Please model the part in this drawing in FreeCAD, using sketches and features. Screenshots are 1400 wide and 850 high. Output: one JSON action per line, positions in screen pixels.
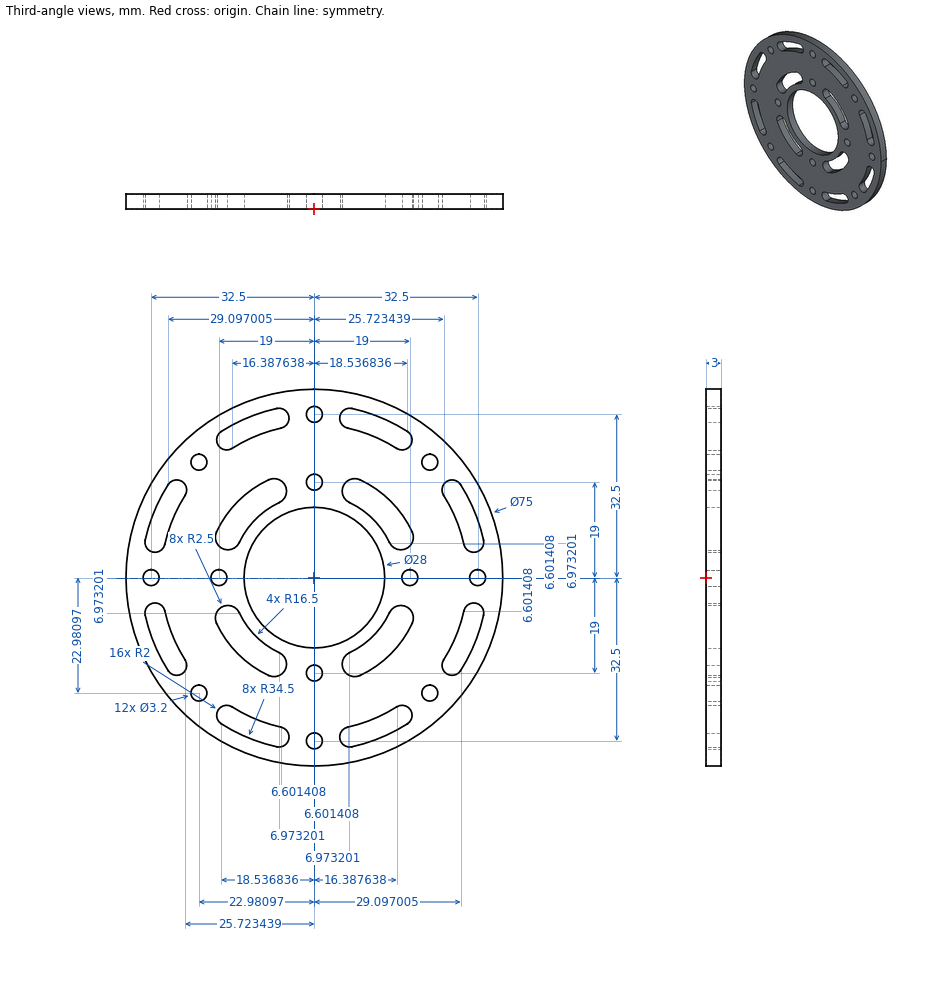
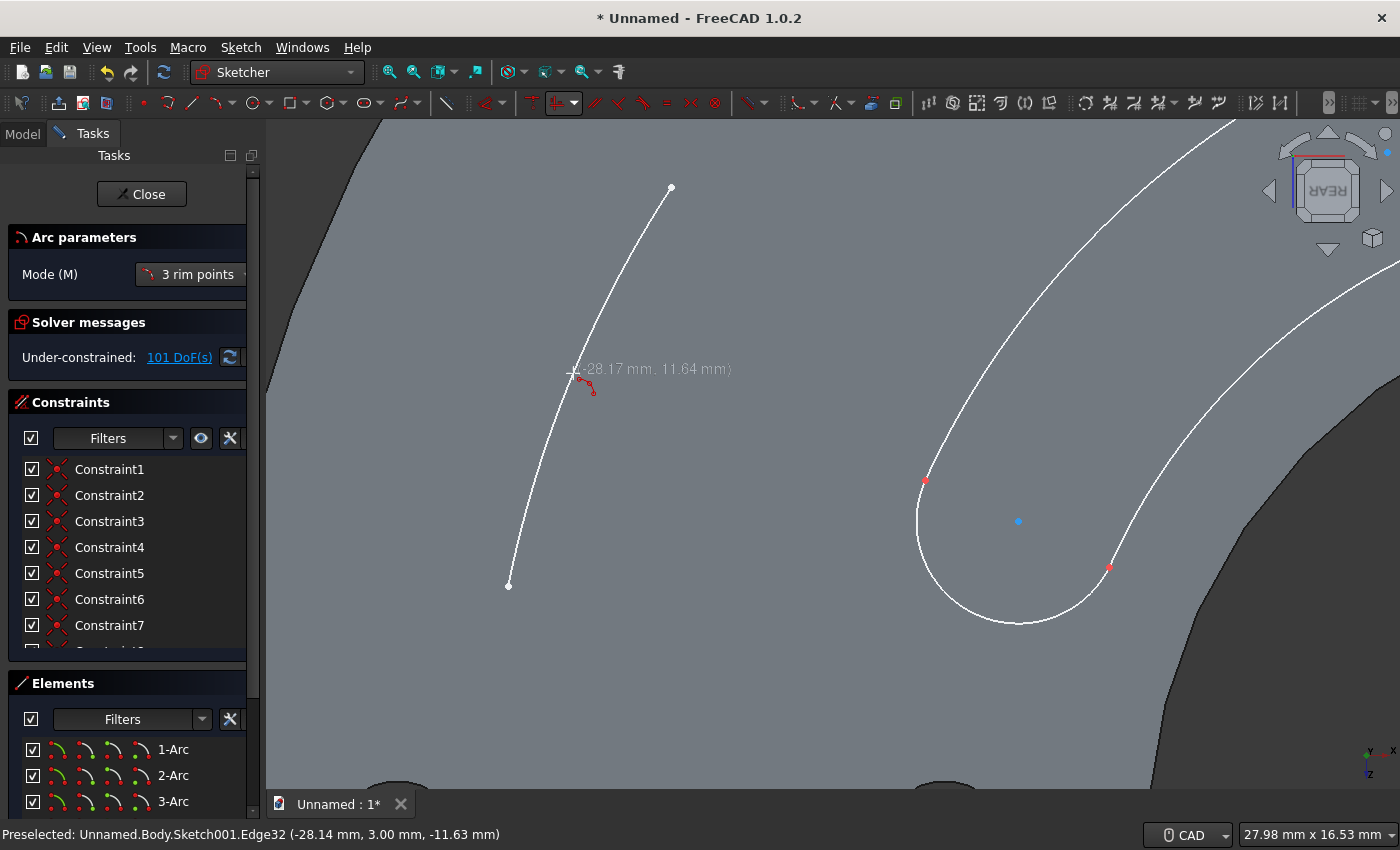
{"action": "scroll", "coordinate": [576, 376], "scroll_direction": "down", "scroll_amount": 9}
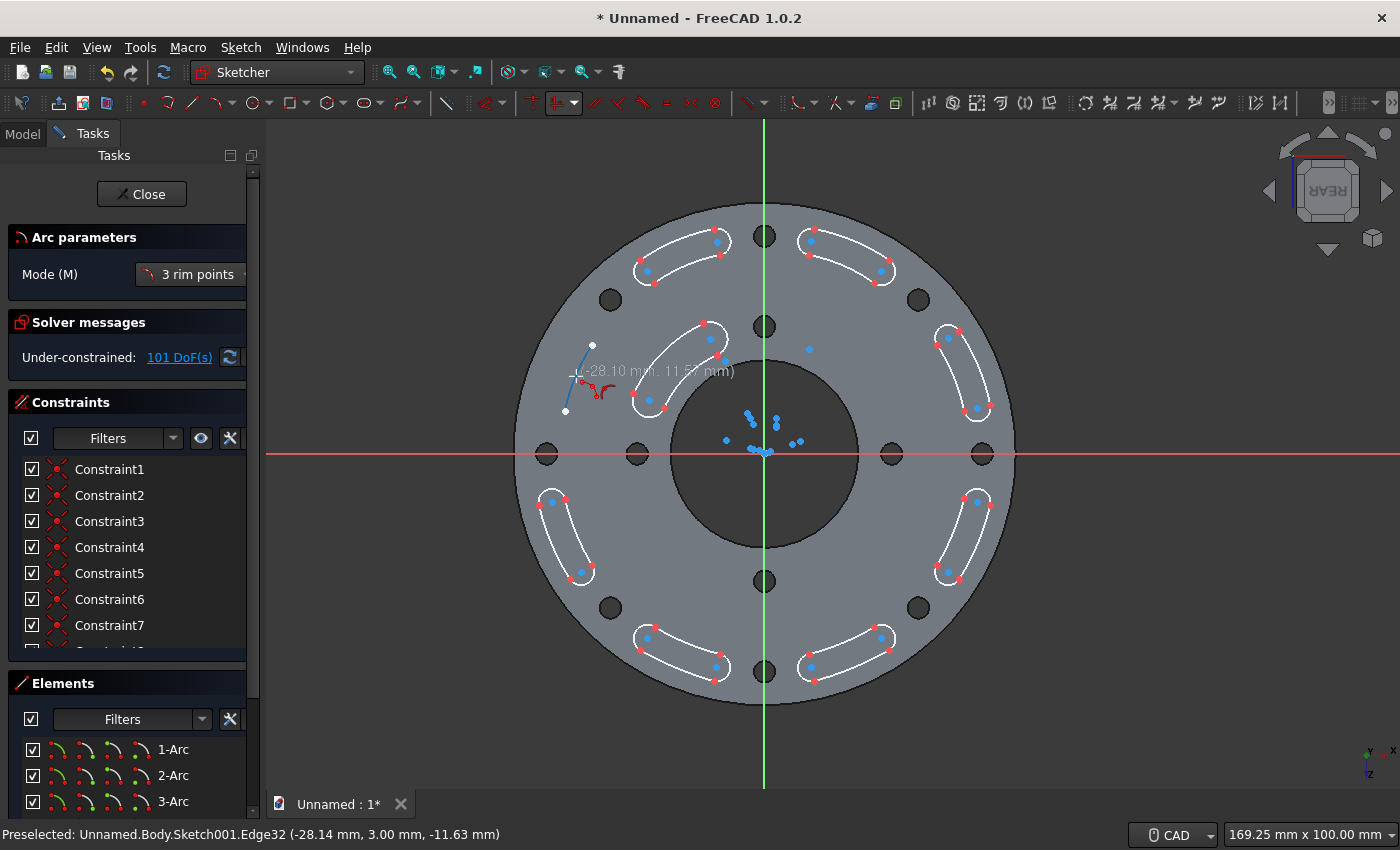
{"action": "left_click", "coordinate": [592, 345]}
{"action": "left_click", "coordinate": [570, 330]}
{"action": "left_click", "coordinate": [588, 326]}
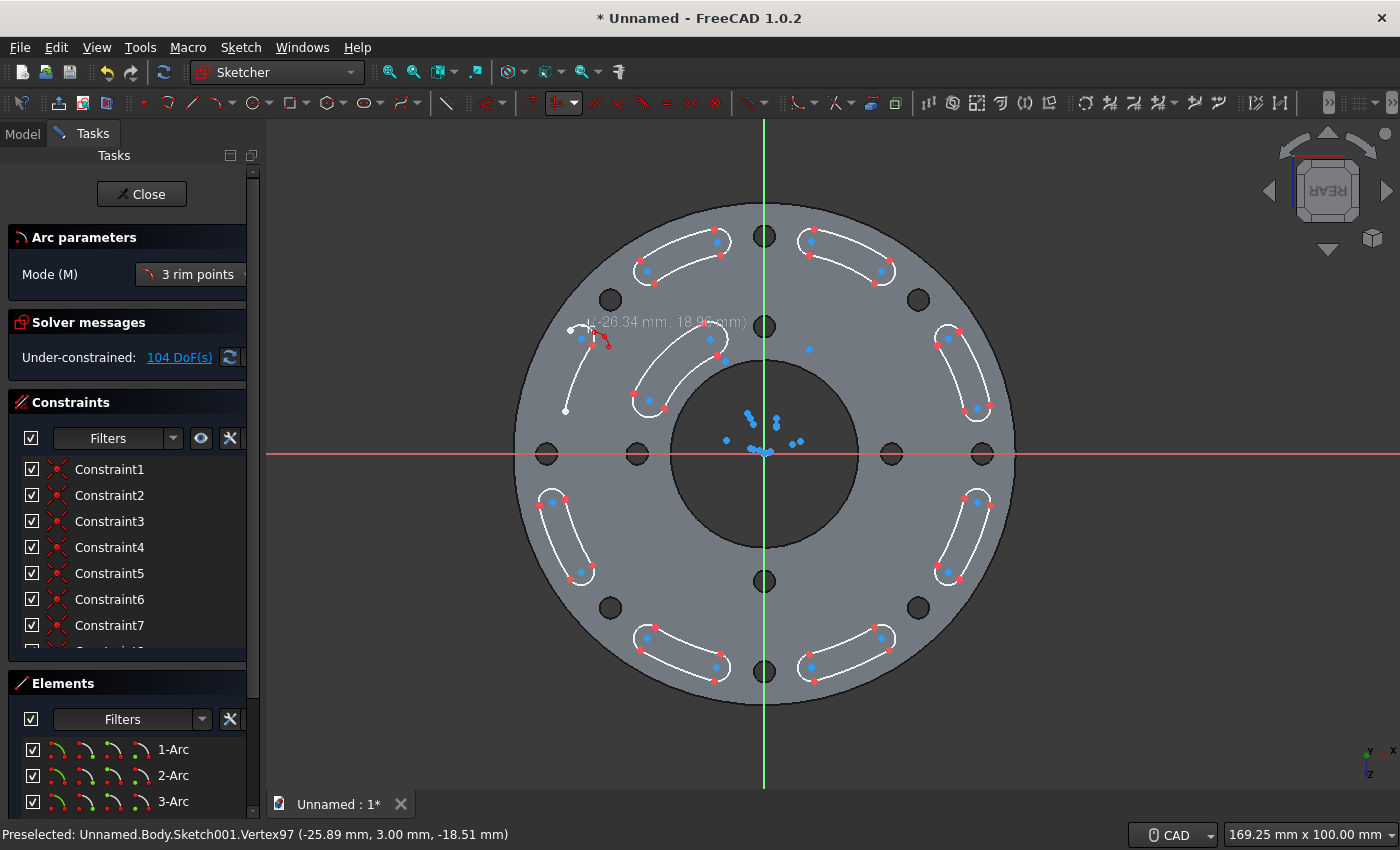
{"action": "left_click", "coordinate": [570, 331]}
{"action": "left_click", "coordinate": [539, 404]}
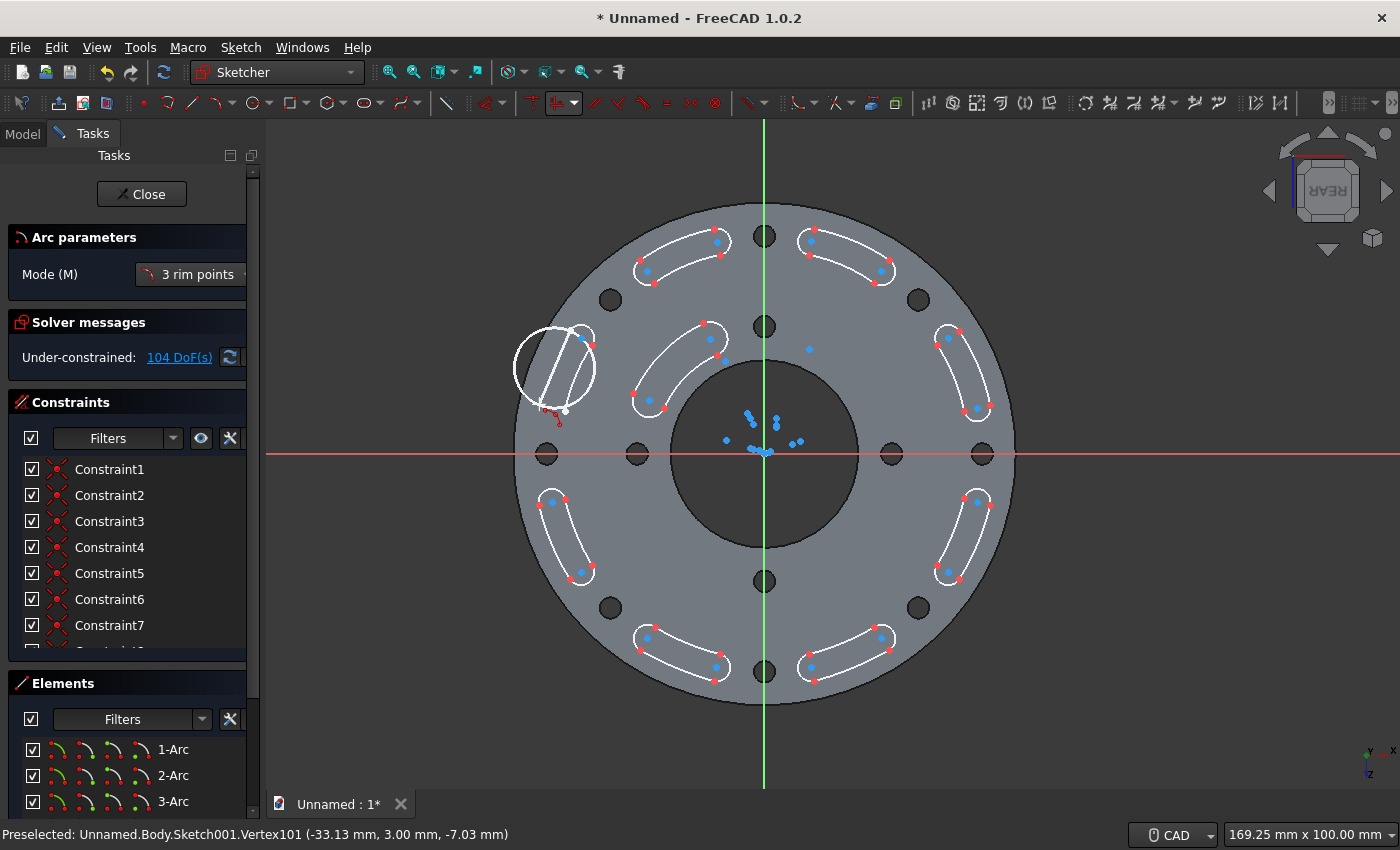
{"action": "scroll", "coordinate": [551, 366], "scroll_direction": "up", "scroll_amount": 8}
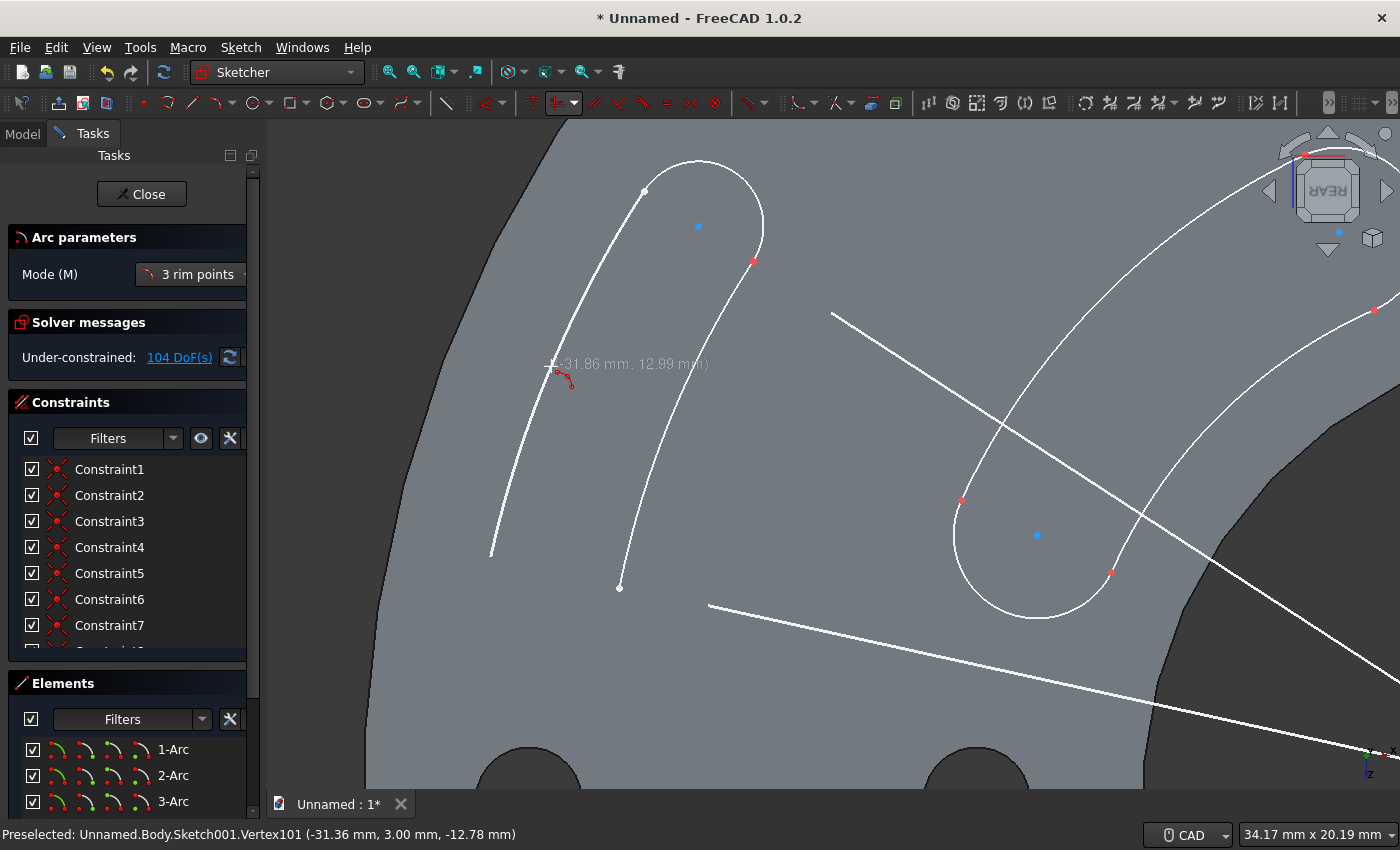
{"action": "left_click", "coordinate": [550, 362]}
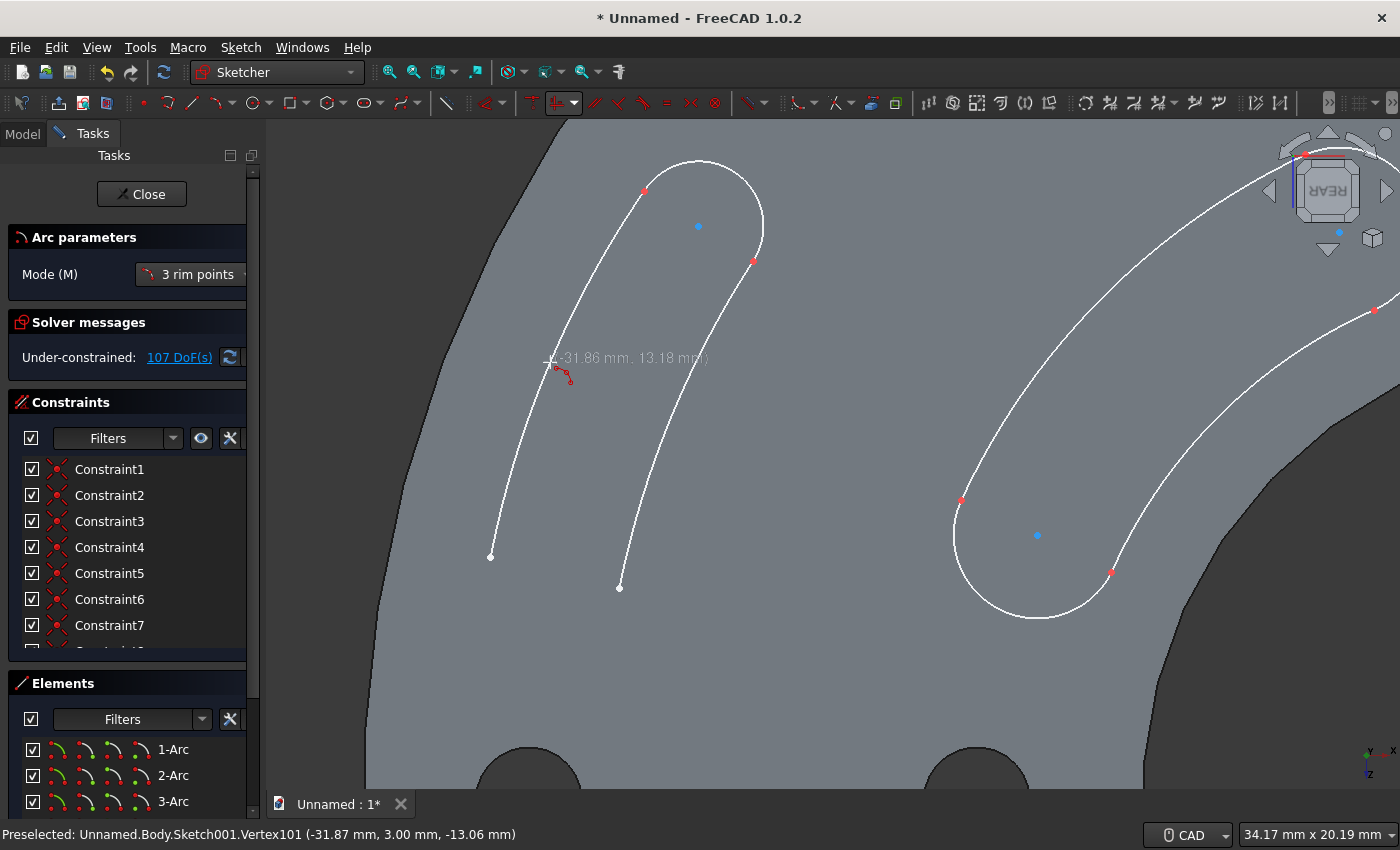
{"action": "scroll", "coordinate": [551, 366], "scroll_direction": "down", "scroll_amount": 8}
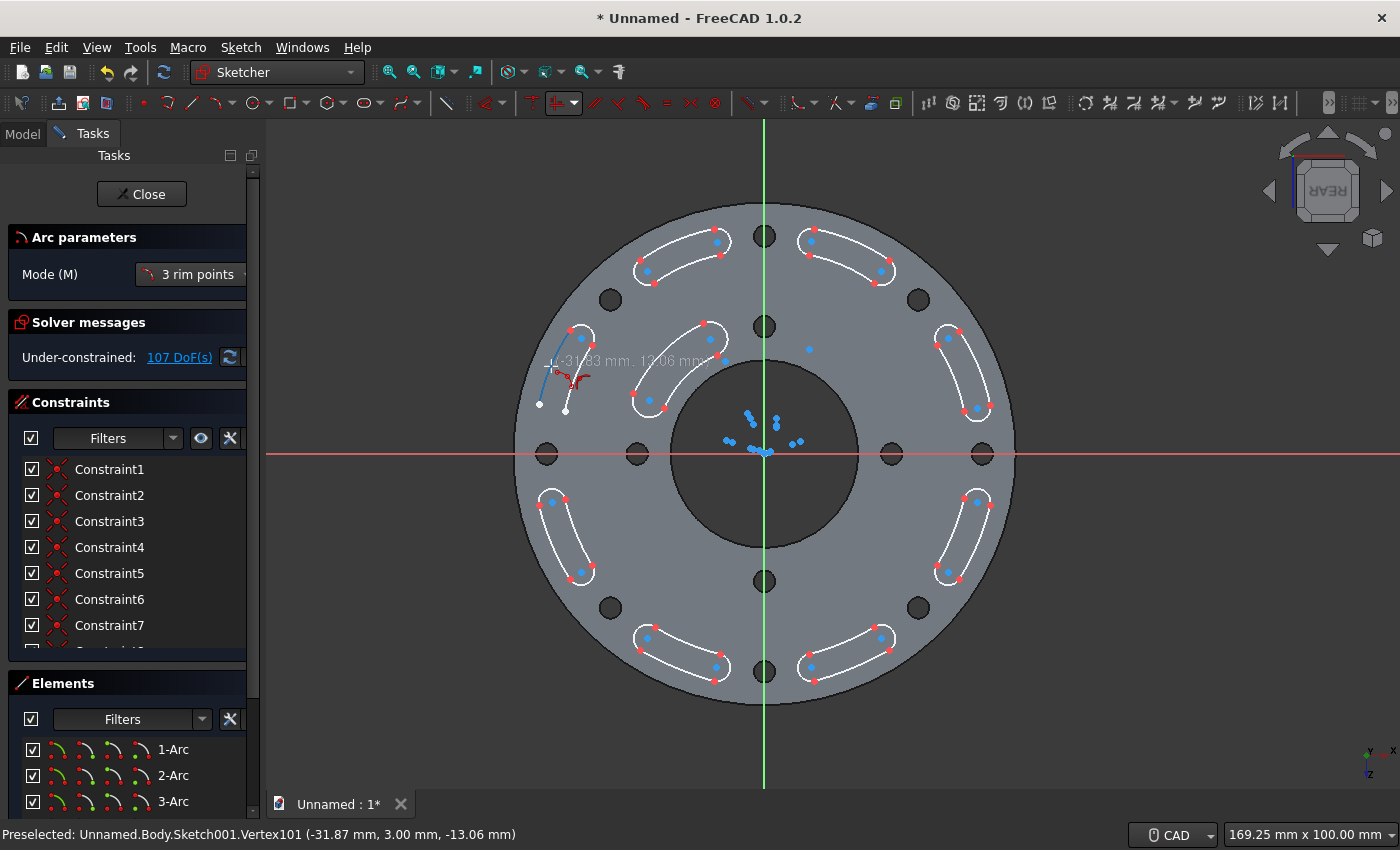
{"action": "left_click", "coordinate": [539, 405]}
{"action": "left_click", "coordinate": [565, 411]}
{"action": "left_click", "coordinate": [549, 420]}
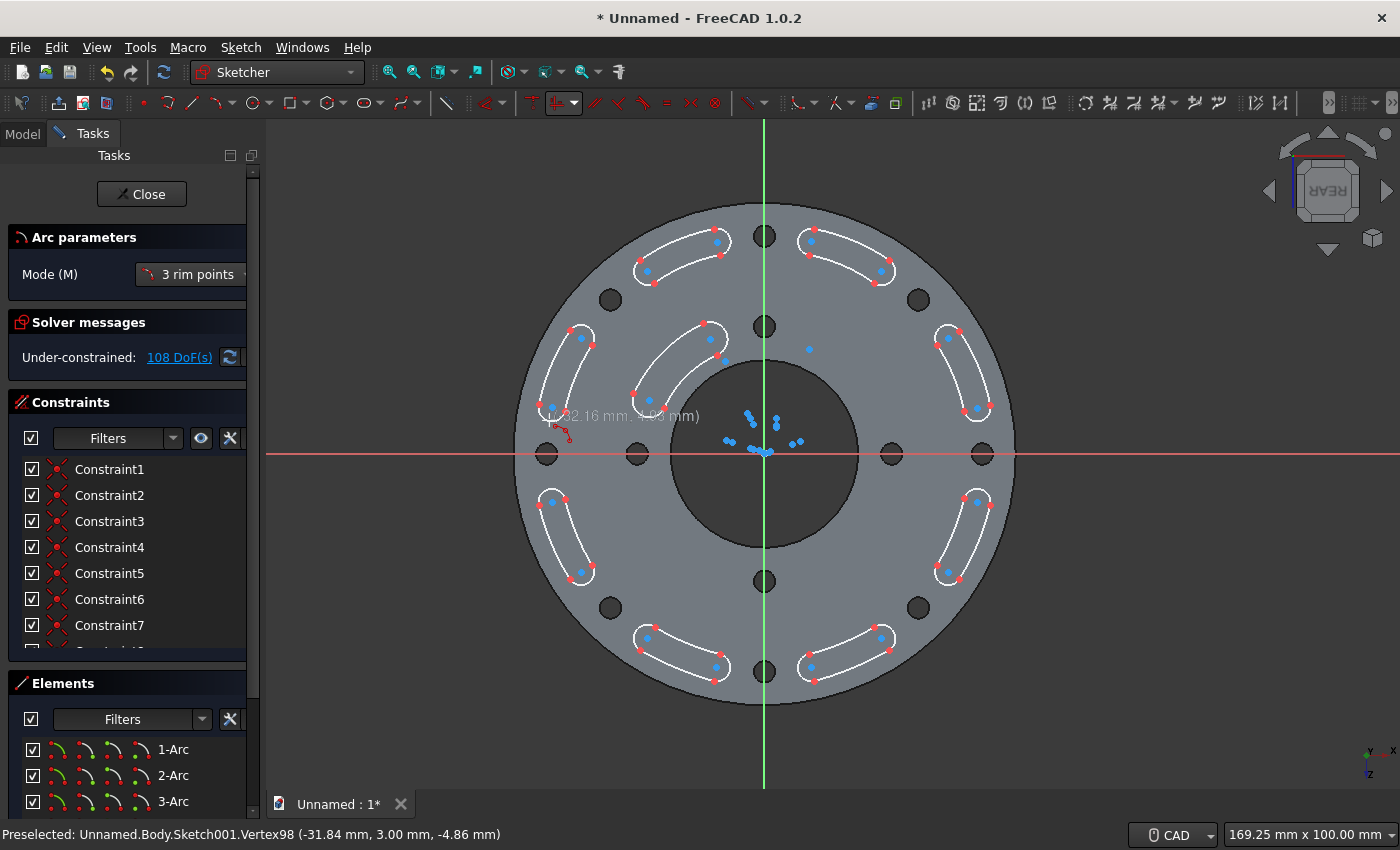
{"action": "left_click", "coordinate": [811, 354]}
{"action": "left_click", "coordinate": [865, 407]}